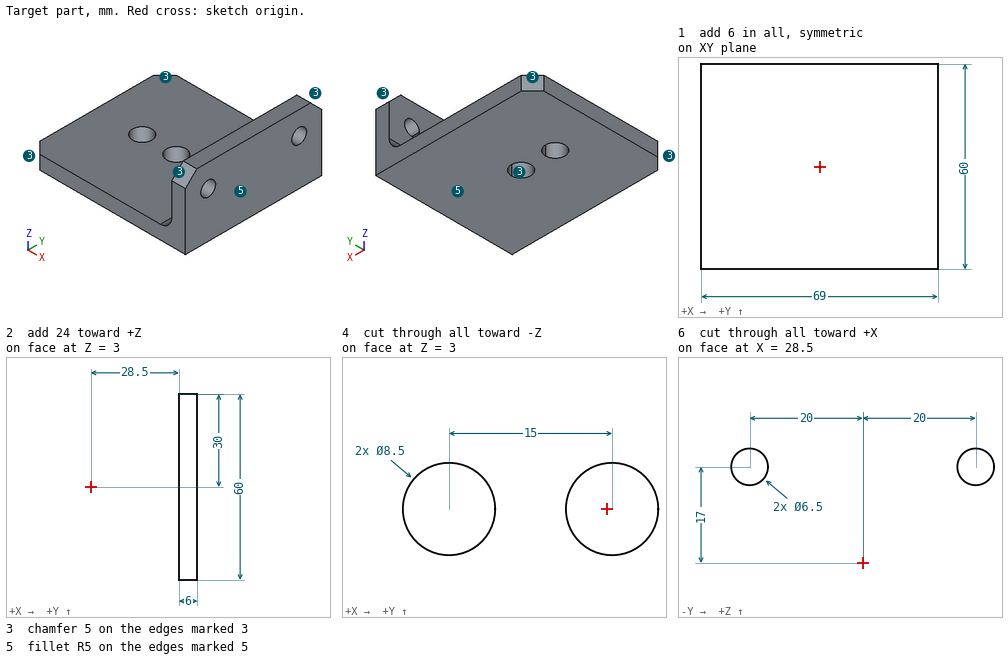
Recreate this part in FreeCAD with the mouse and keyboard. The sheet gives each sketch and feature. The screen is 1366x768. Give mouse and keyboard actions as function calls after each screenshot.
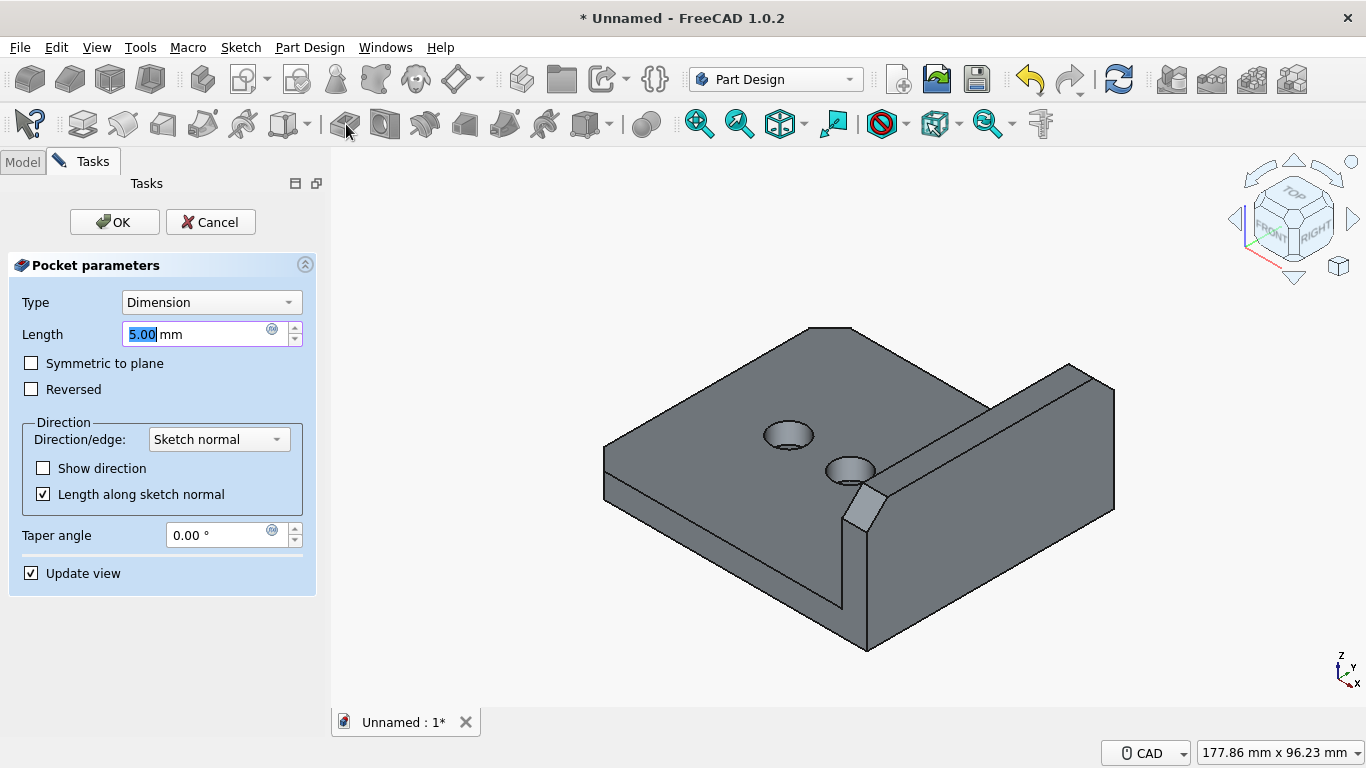
click(212, 302)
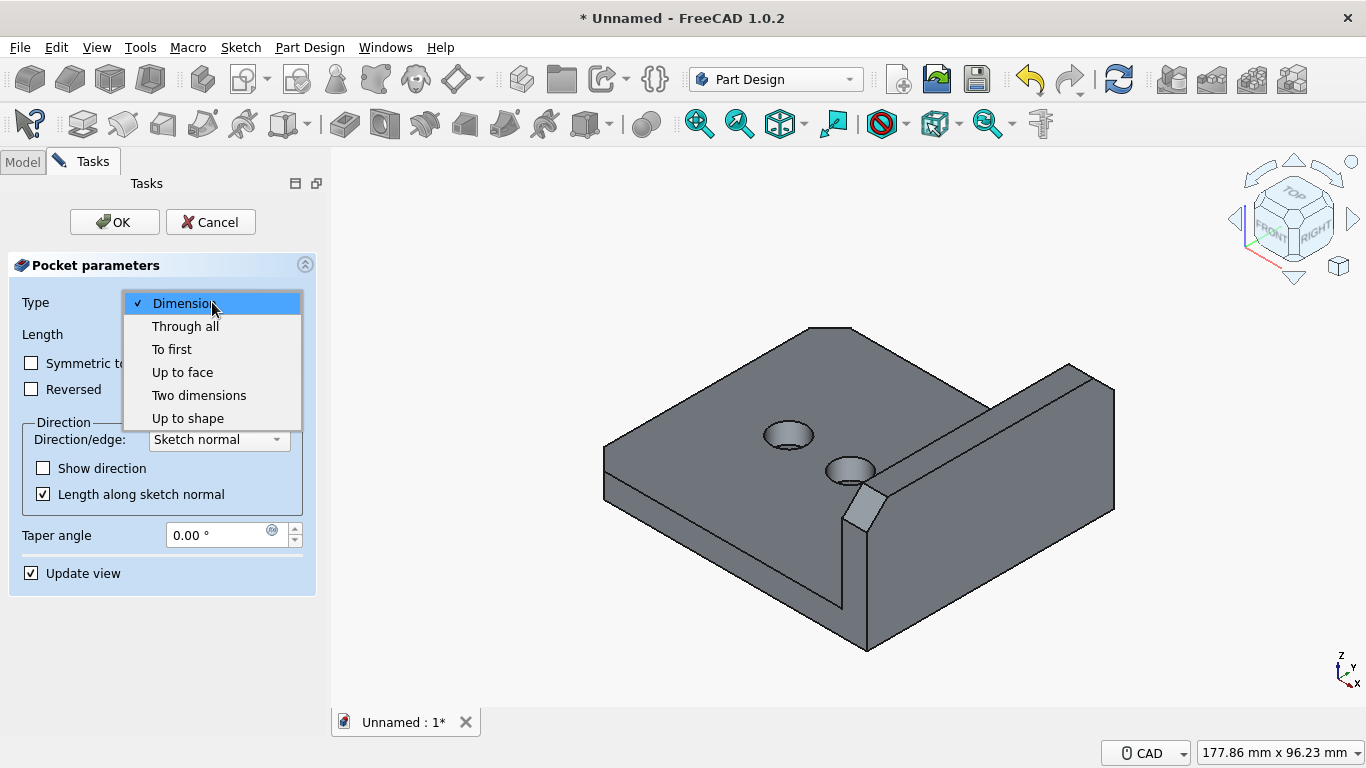
click(212, 326)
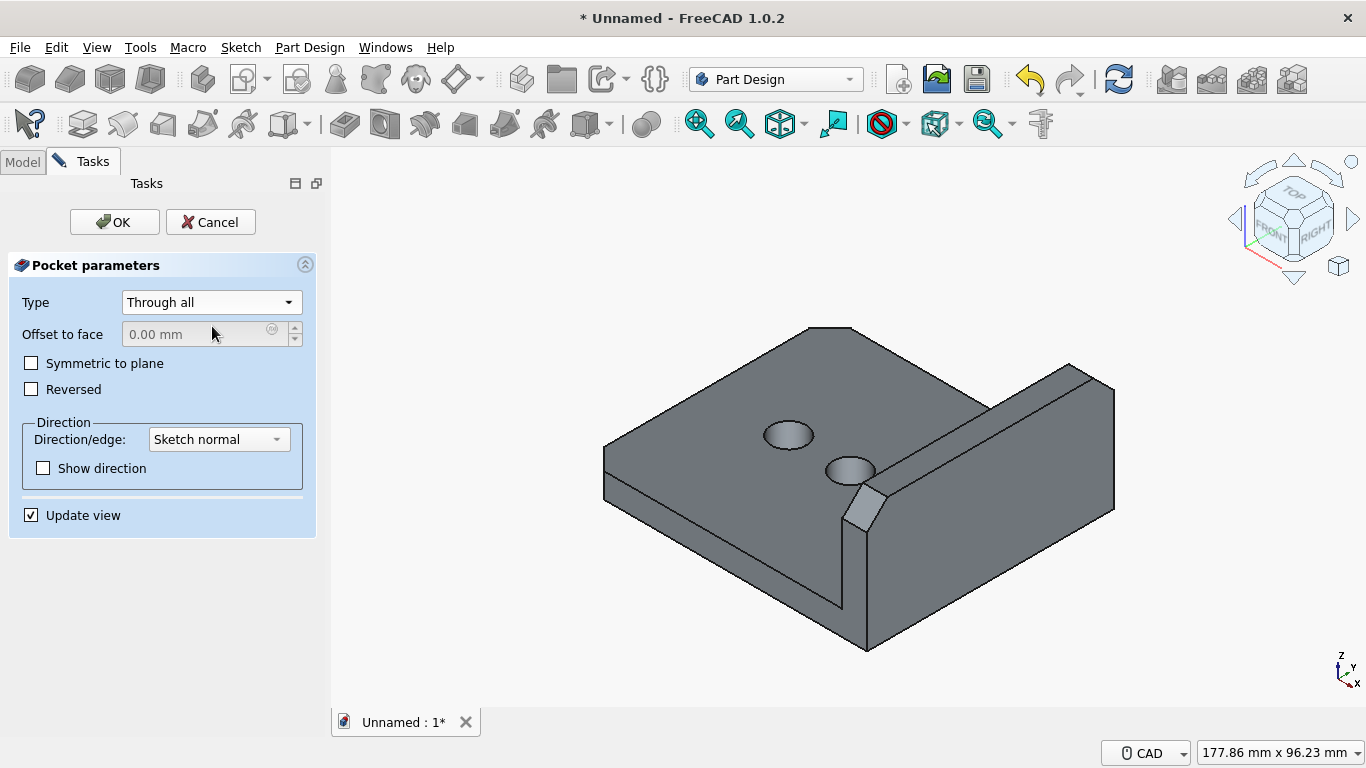
click(115, 222)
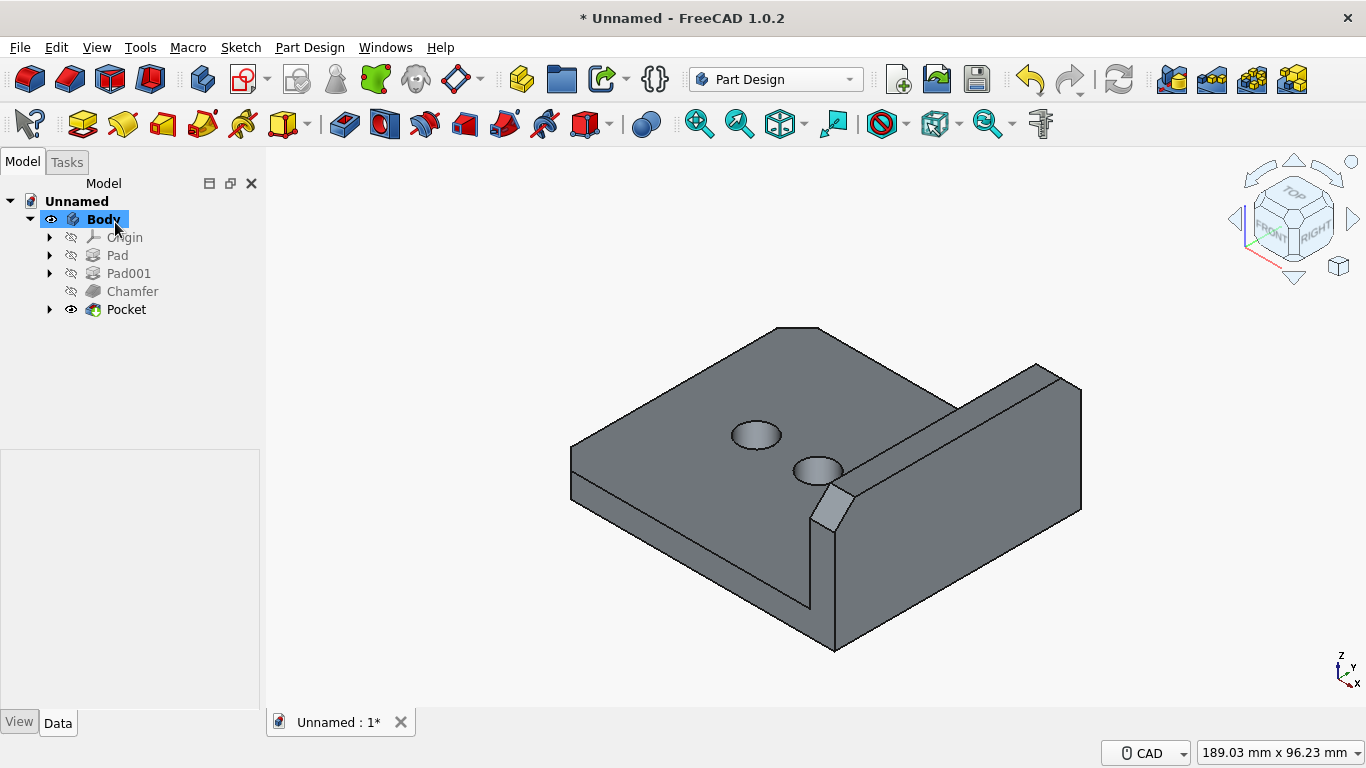
key(2)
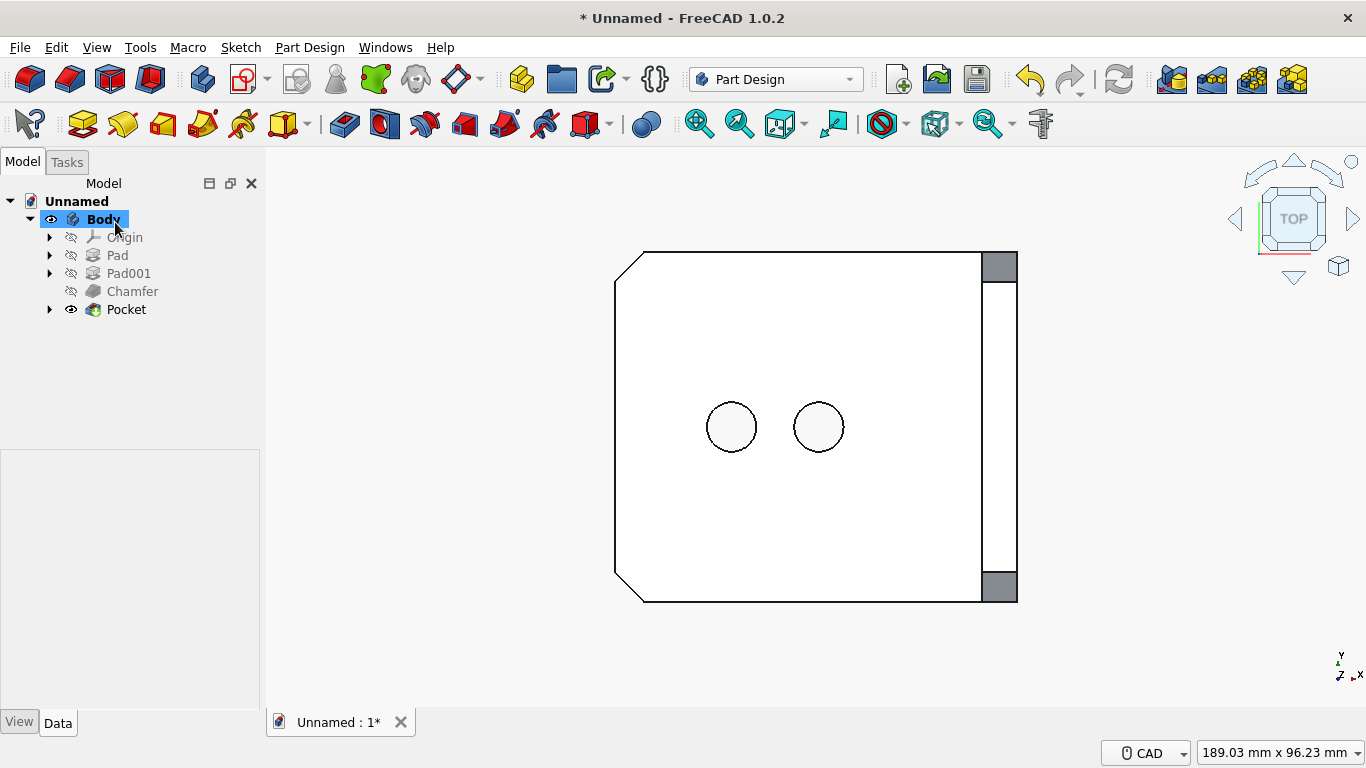
key(0)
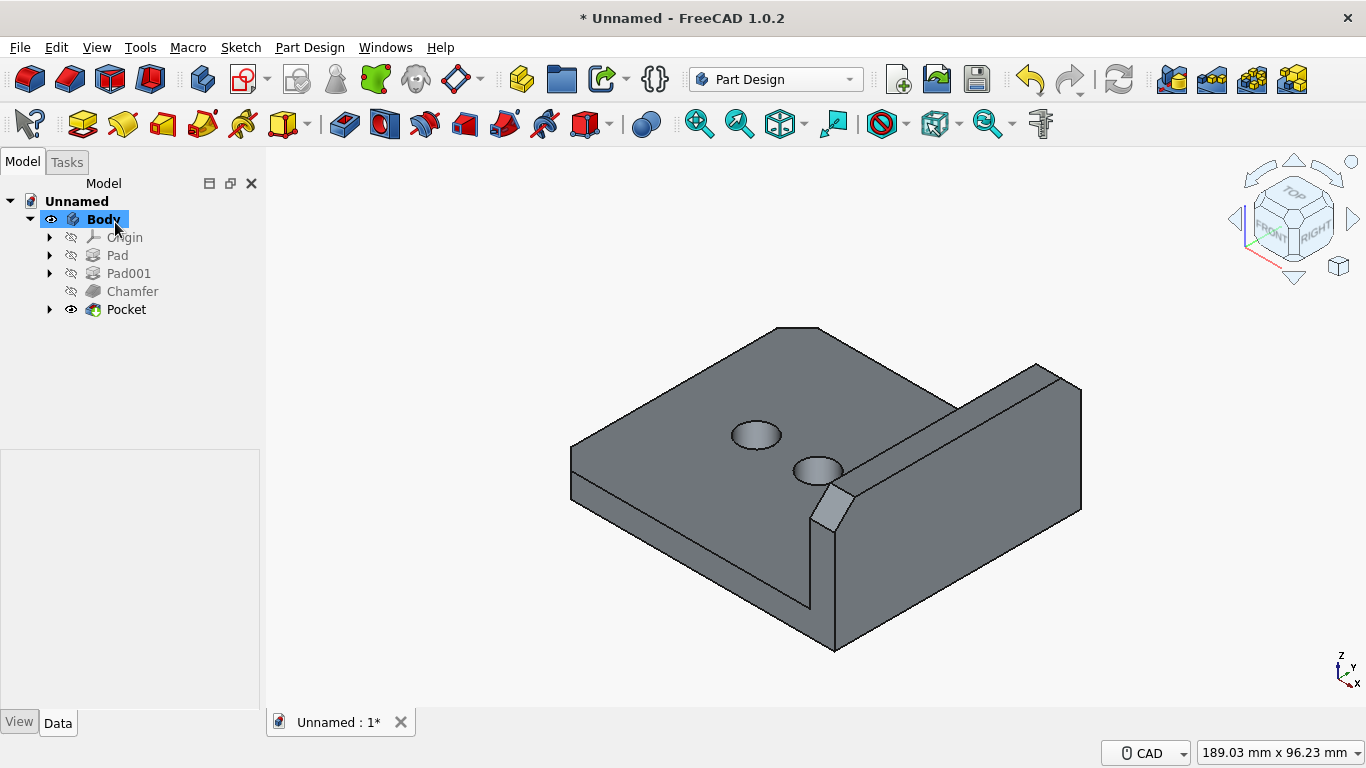
key(1)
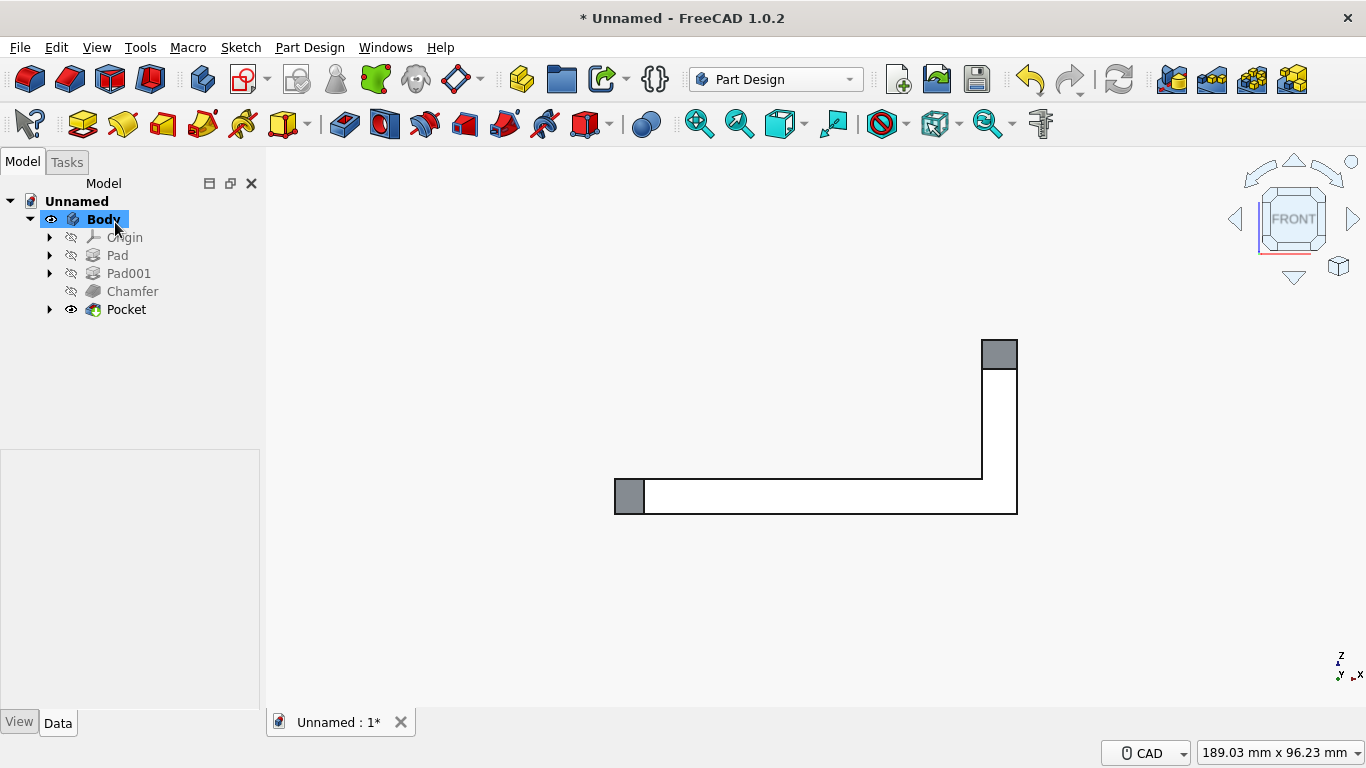
click(700, 124)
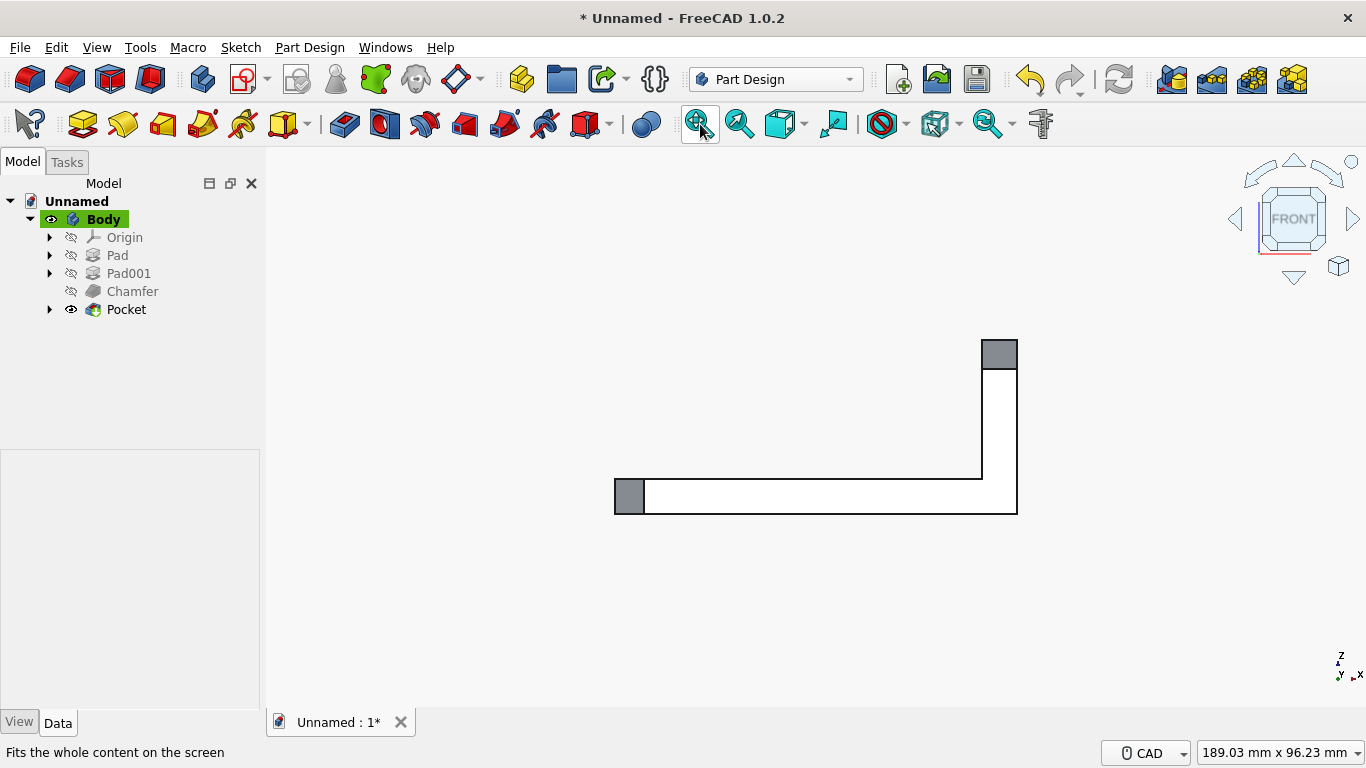
key(3)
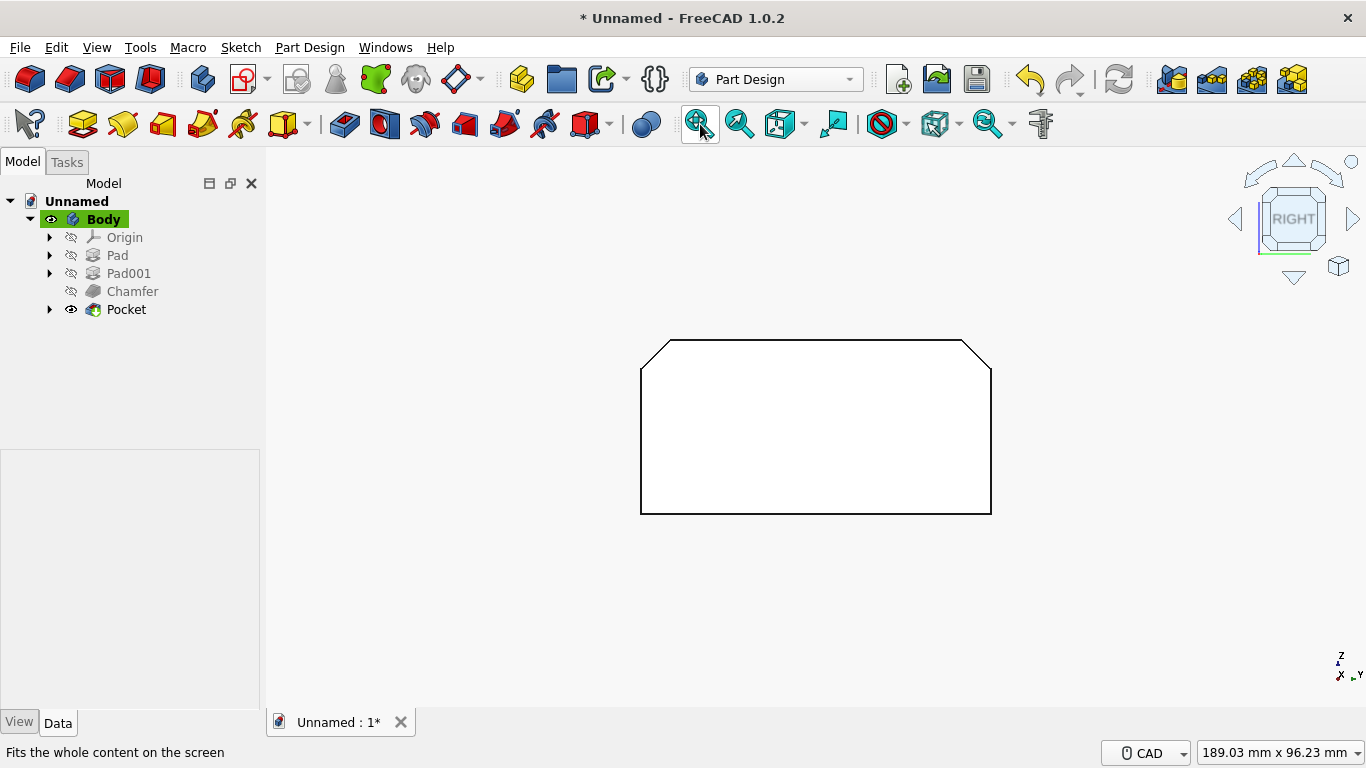
click(700, 124)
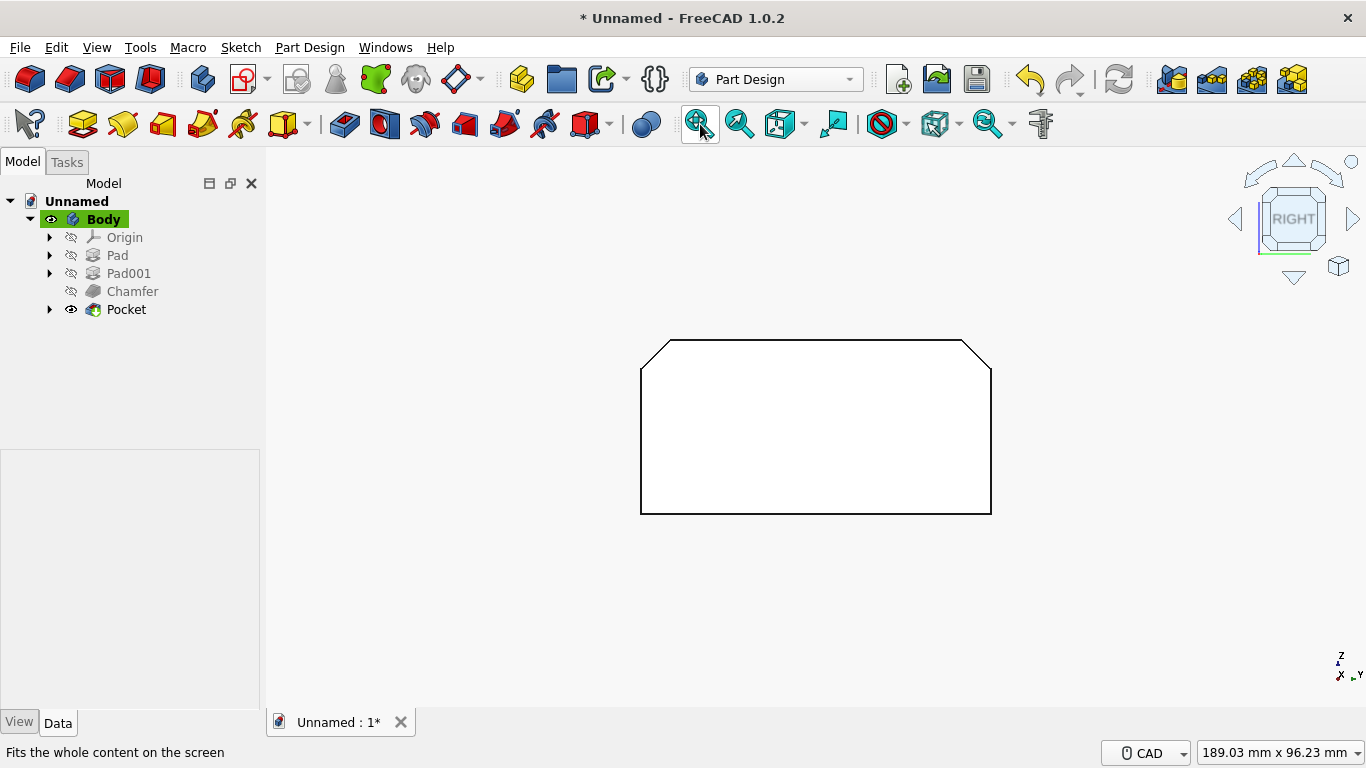
key(5)